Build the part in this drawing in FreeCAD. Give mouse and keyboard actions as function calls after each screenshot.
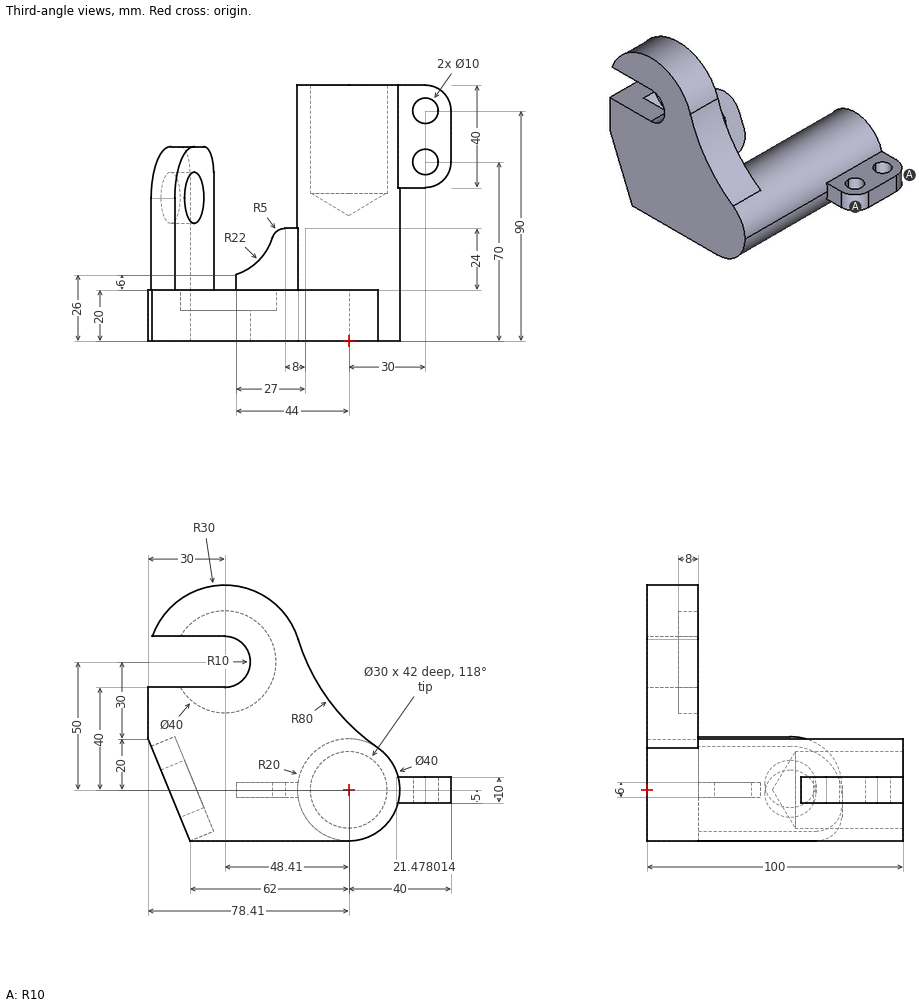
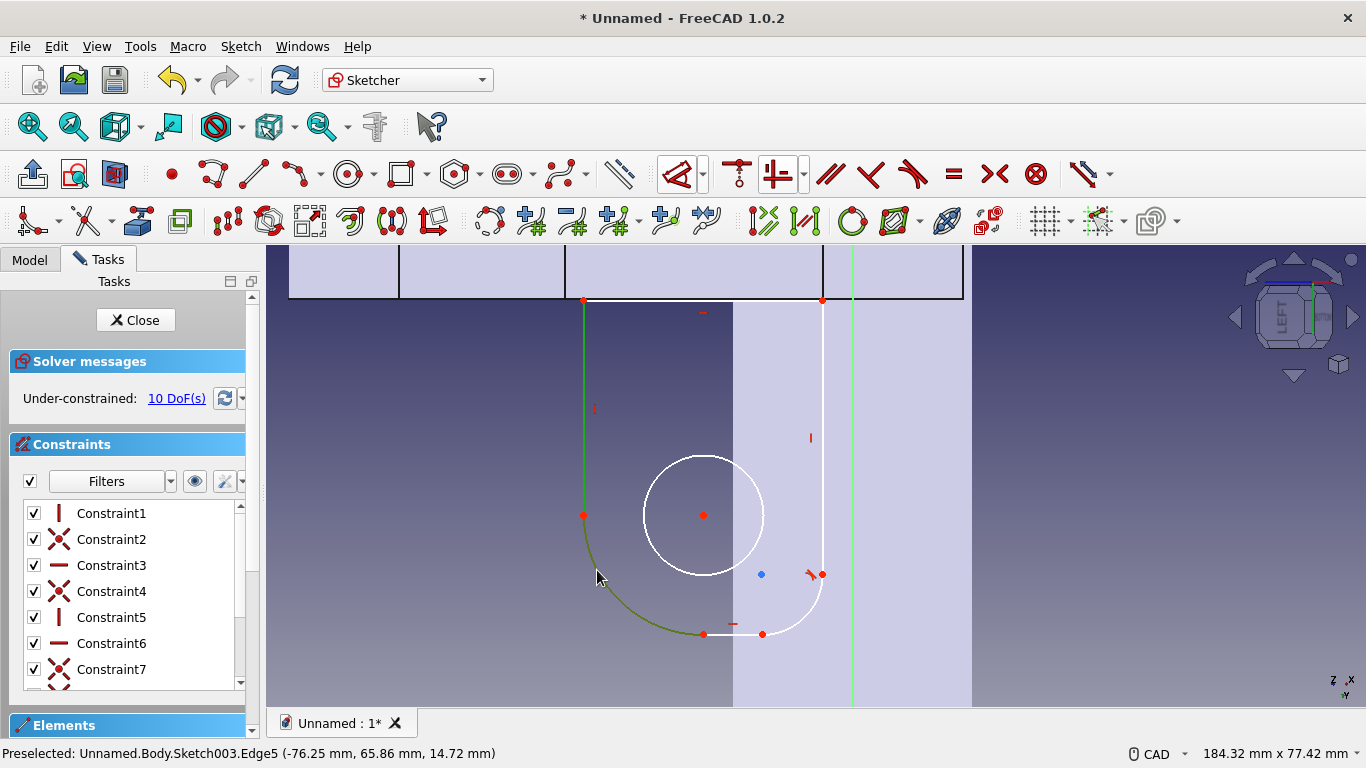
key(t)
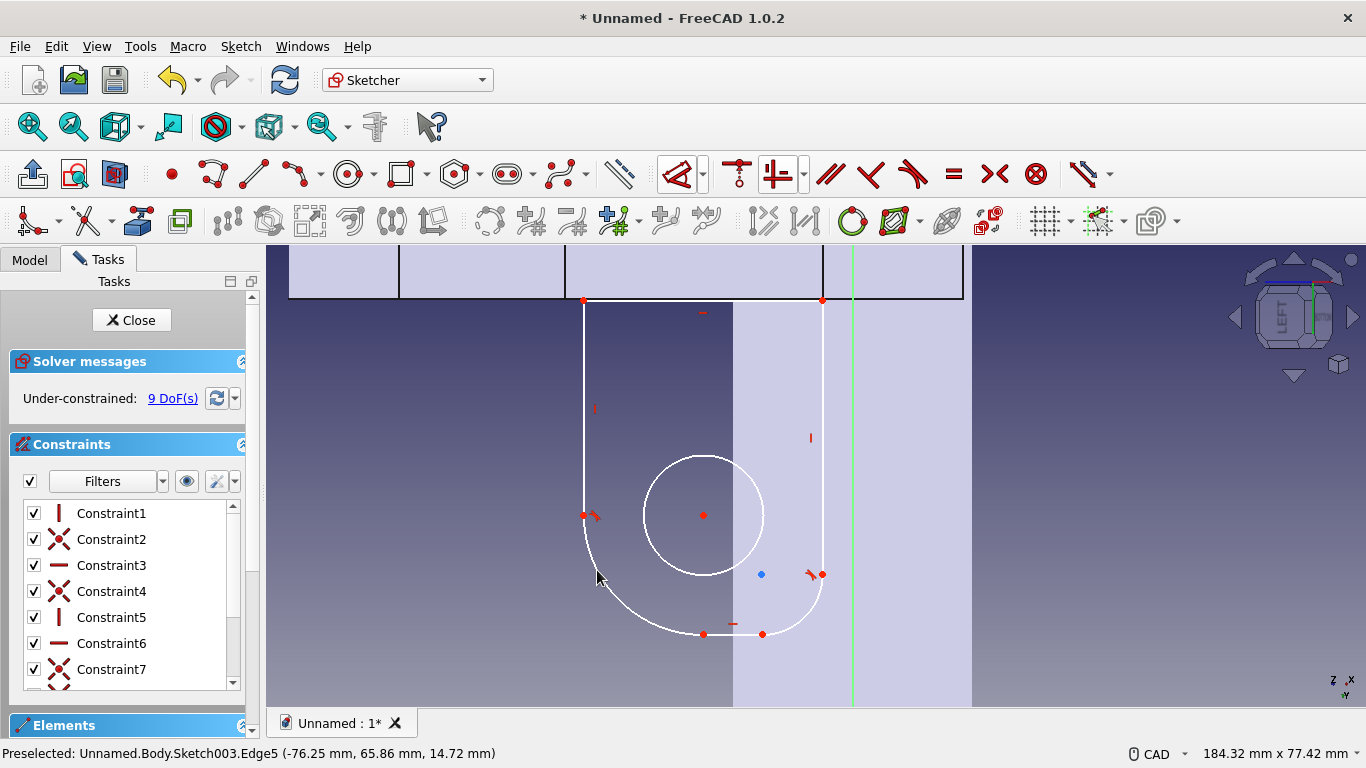
click(721, 635)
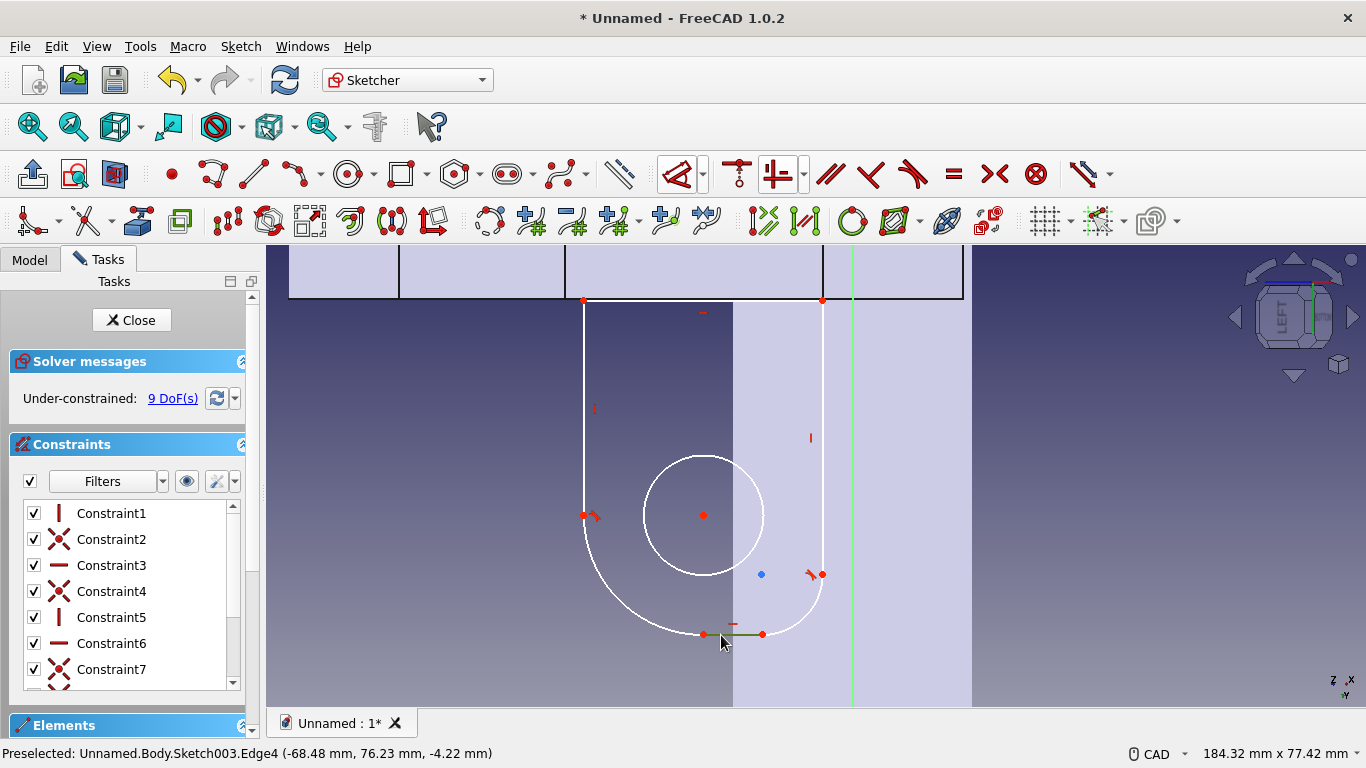
click(597, 570)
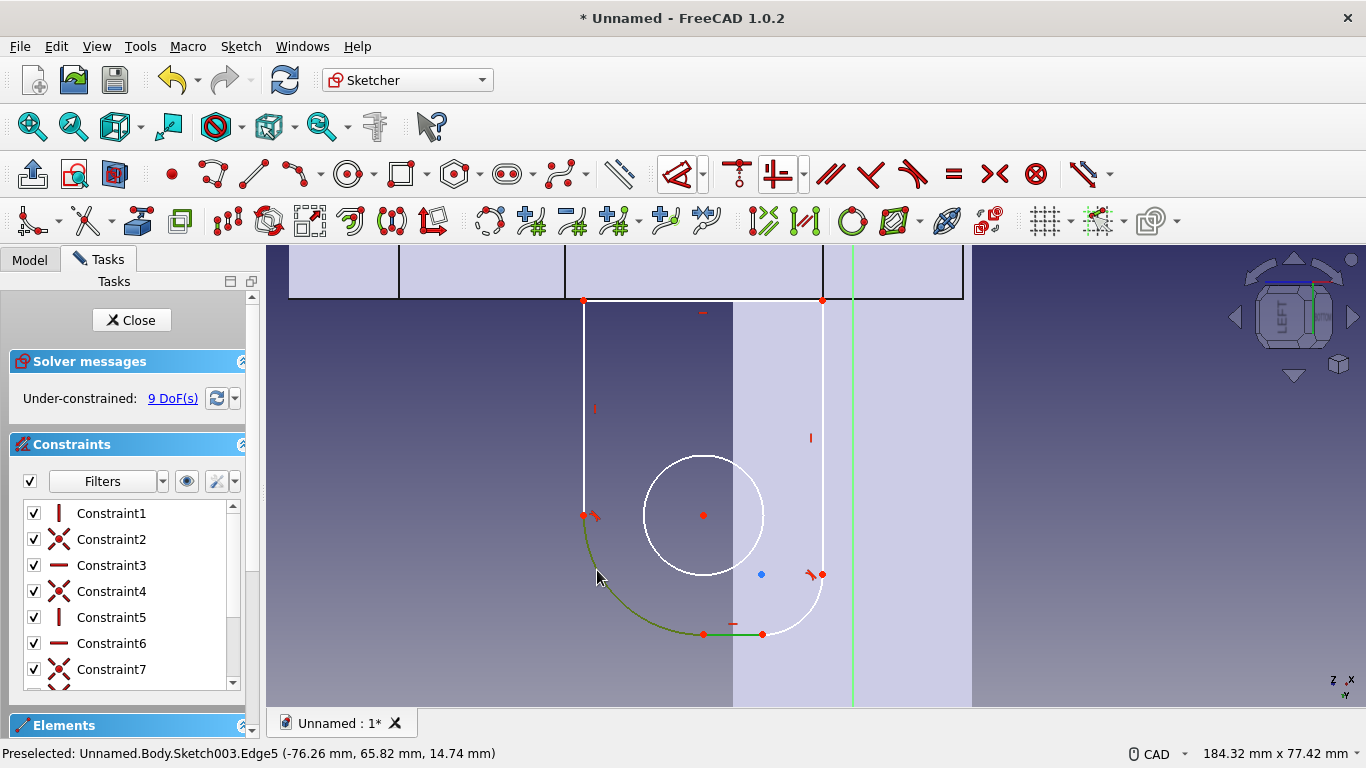
key(t)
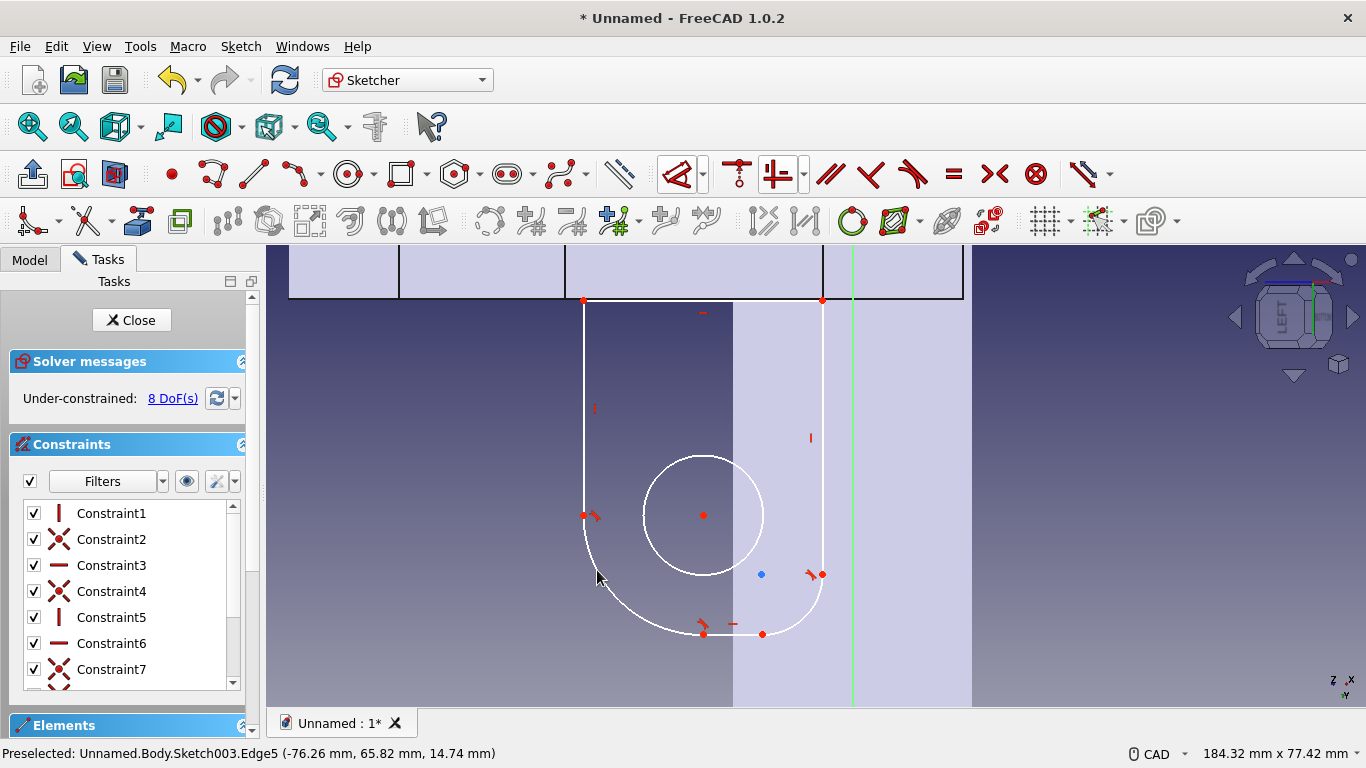
click(721, 635)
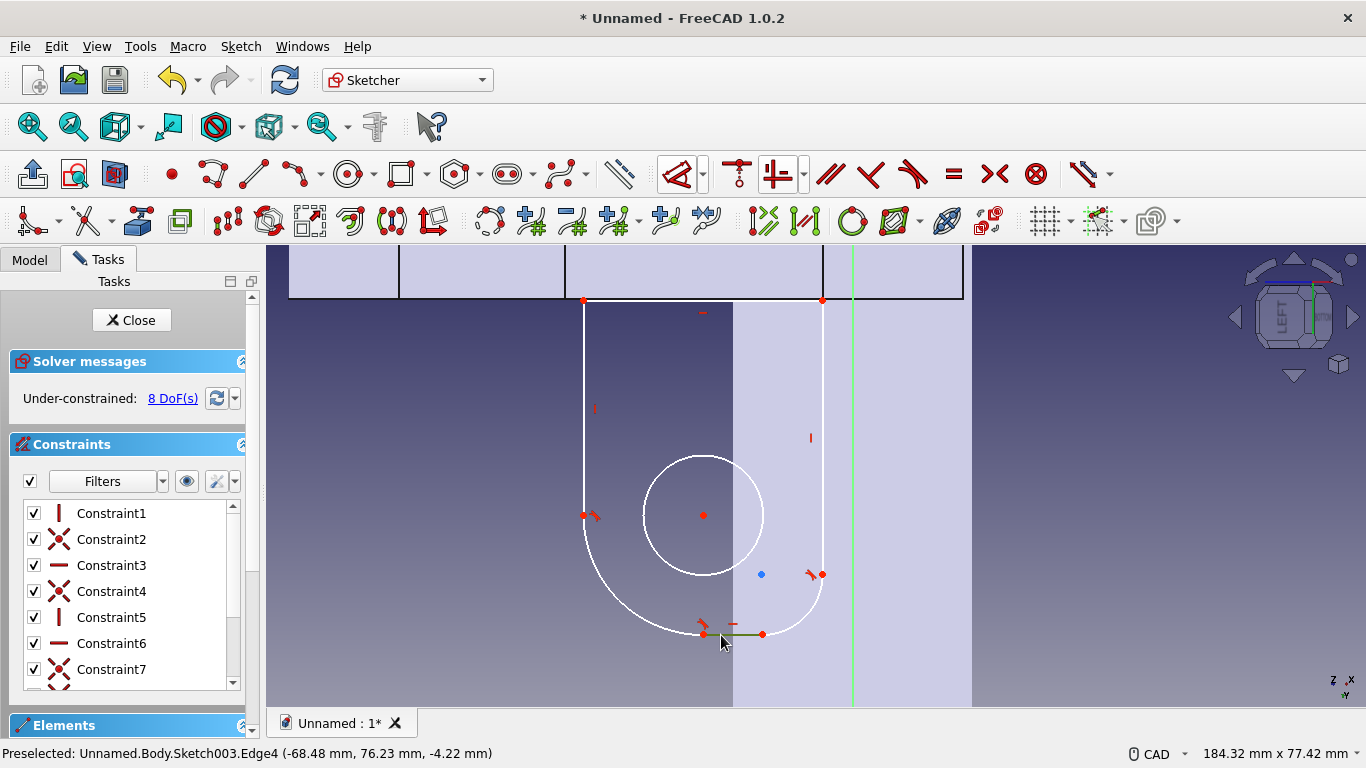
click(790, 628)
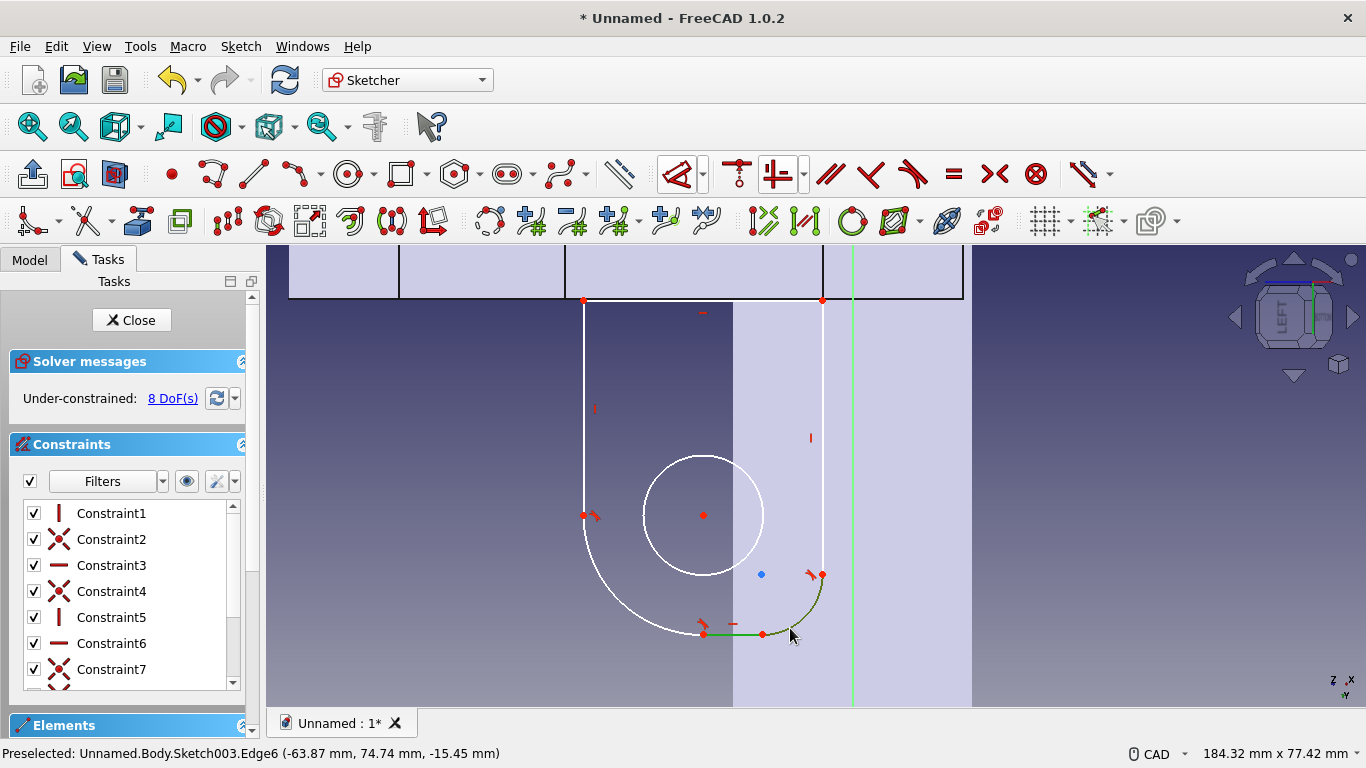
key(t)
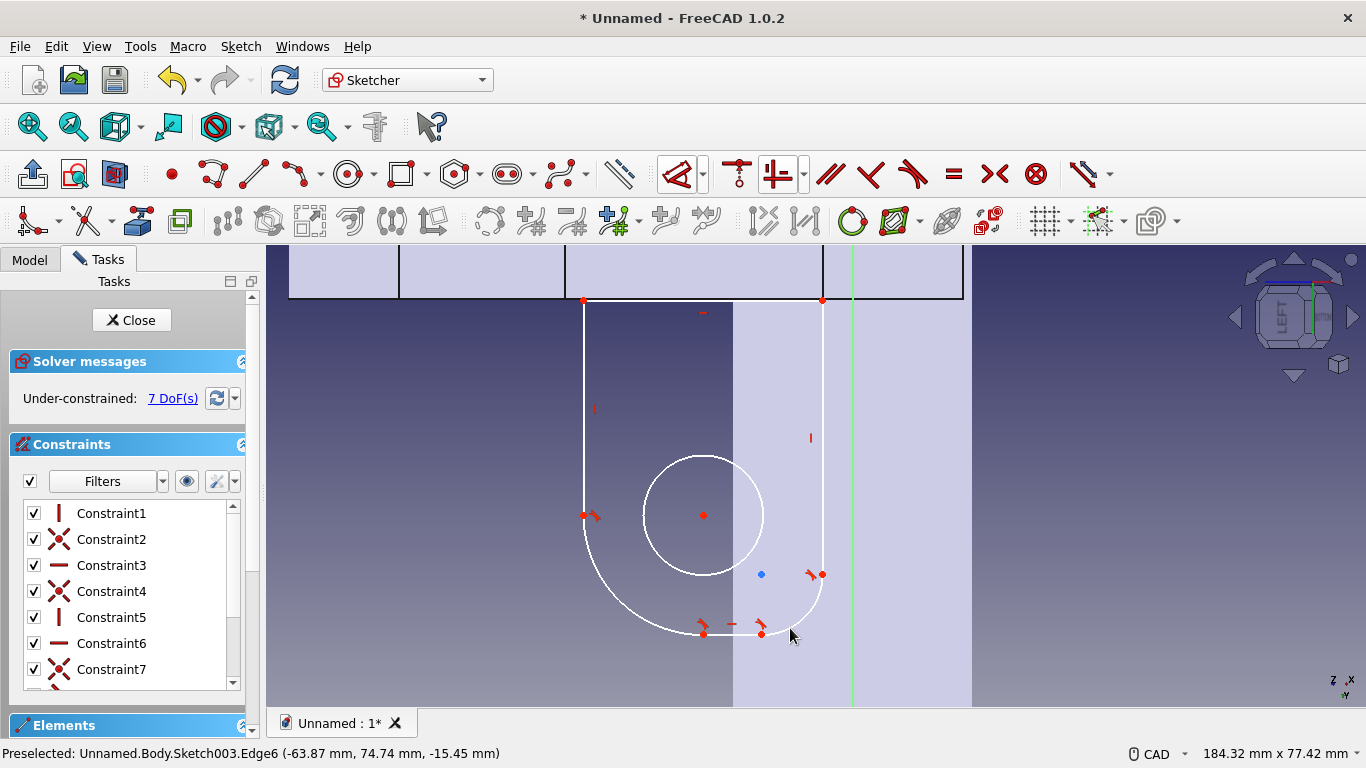
key(d)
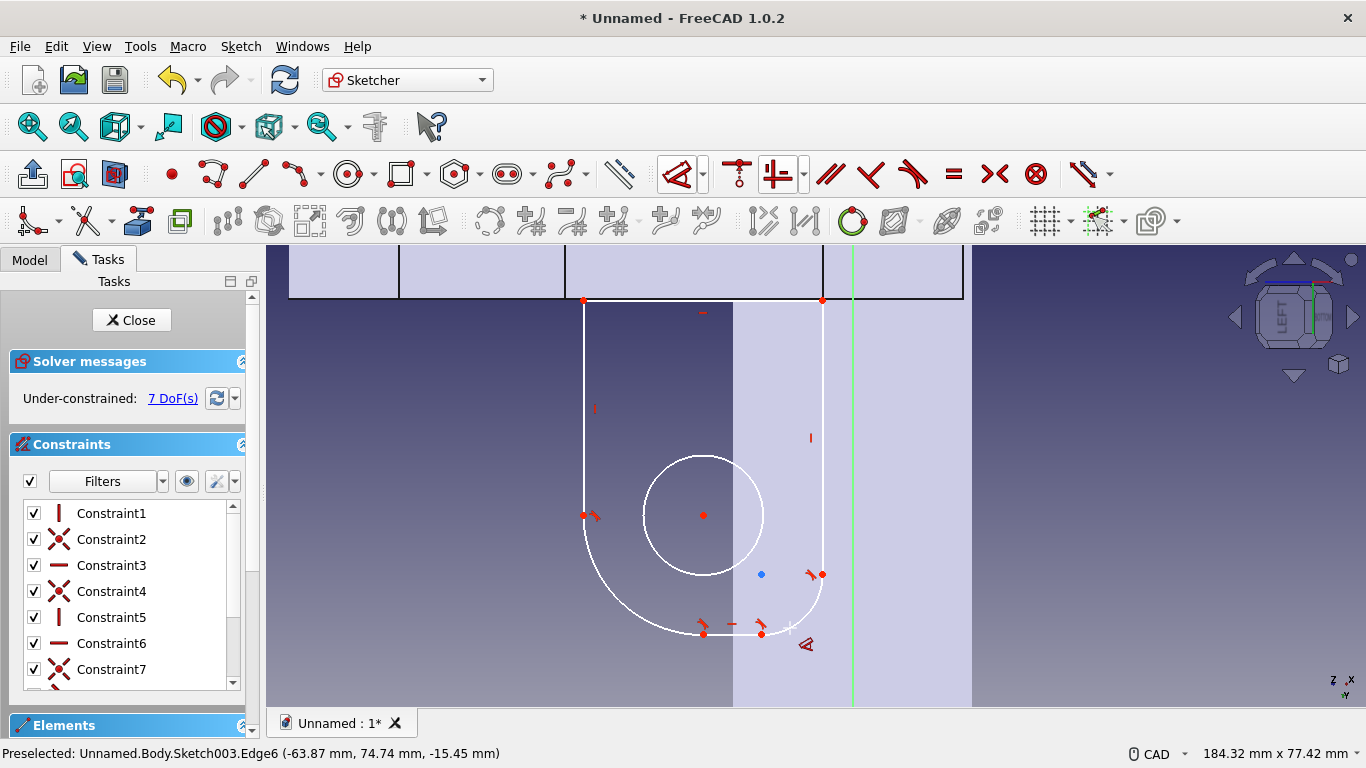
click(597, 570)
click(569, 585)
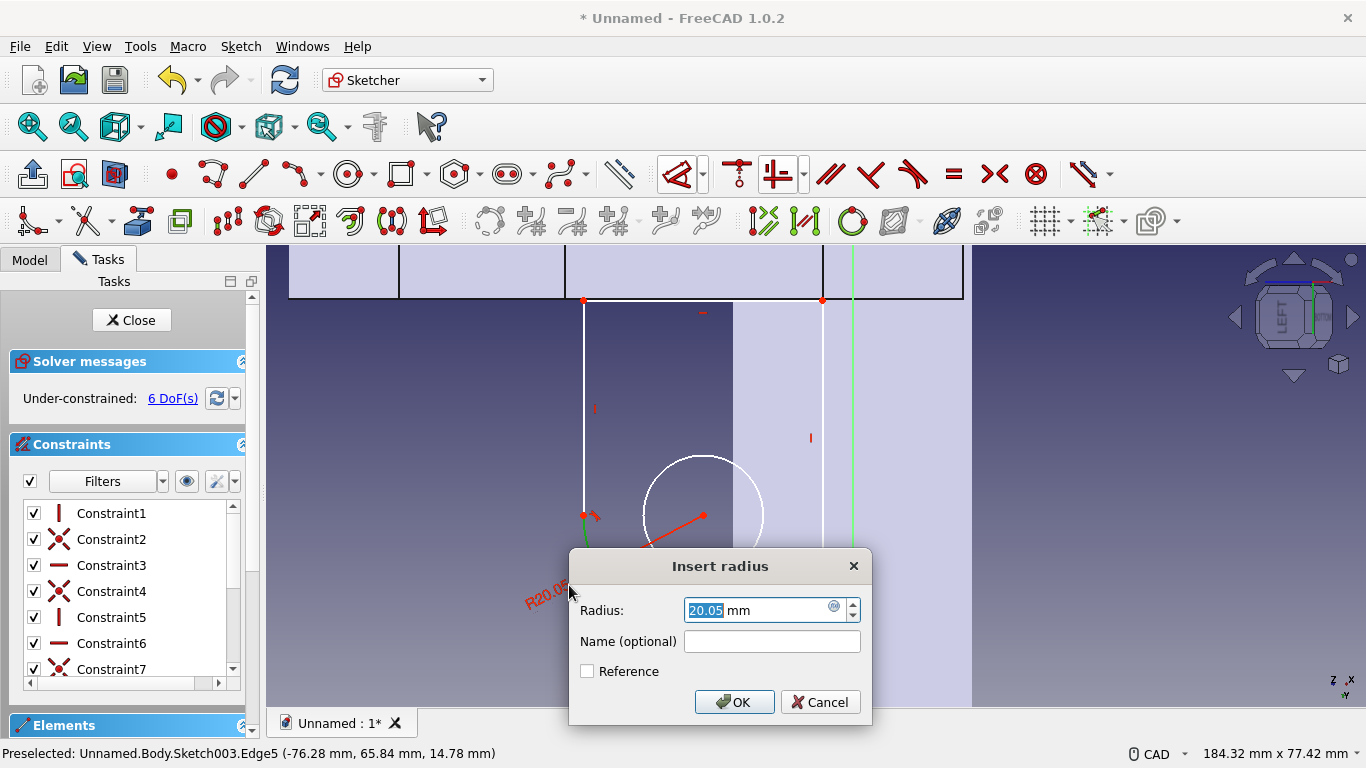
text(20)
key(Return)